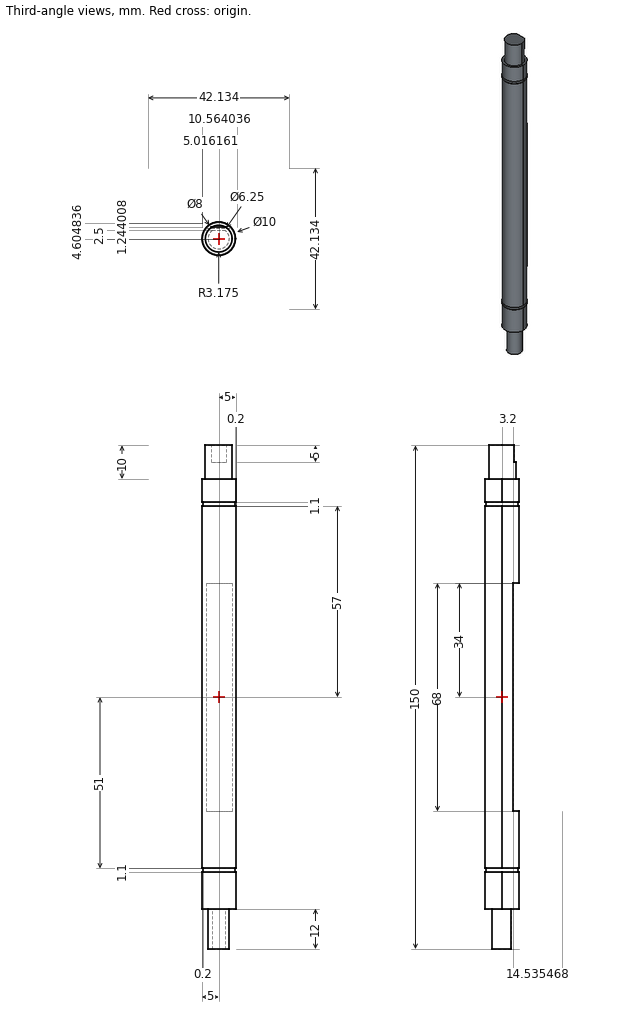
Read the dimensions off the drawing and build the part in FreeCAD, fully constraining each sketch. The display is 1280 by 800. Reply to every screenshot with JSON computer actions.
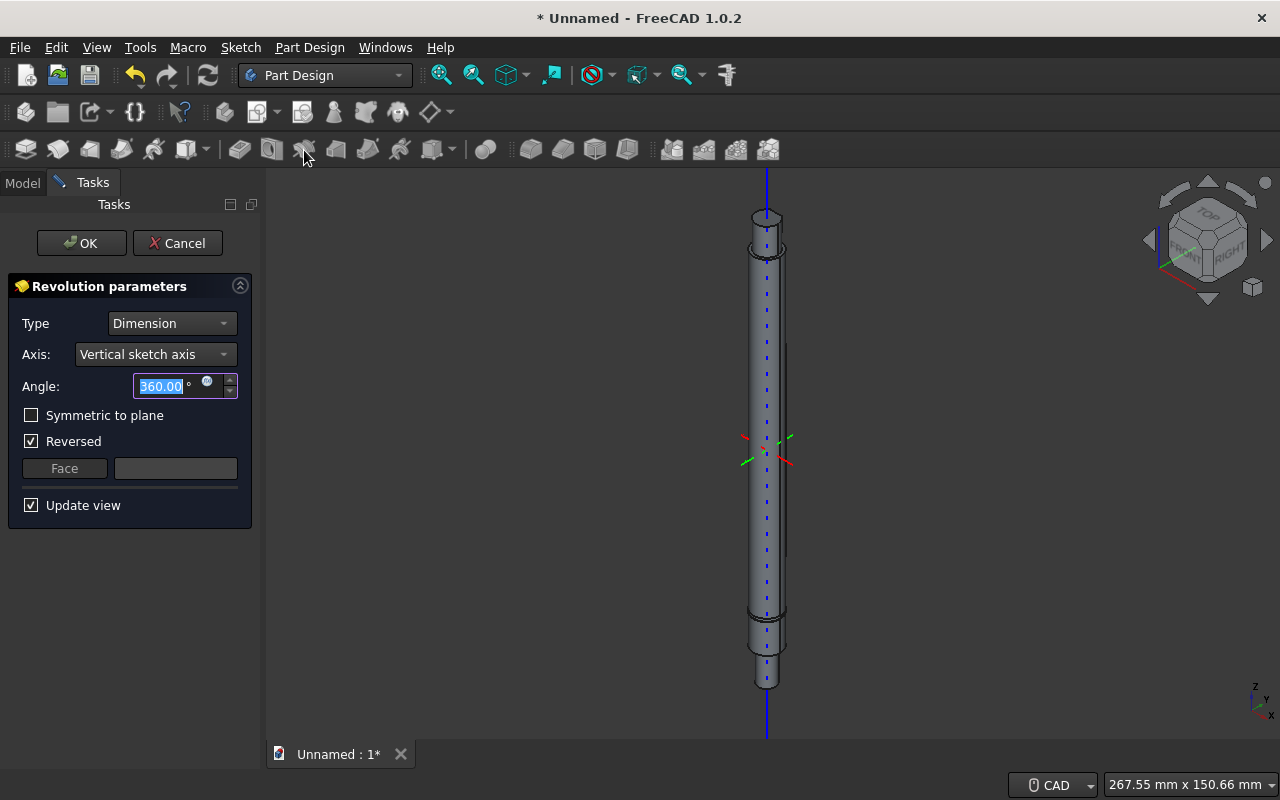
{"action": "left_click", "coordinate": [82, 243]}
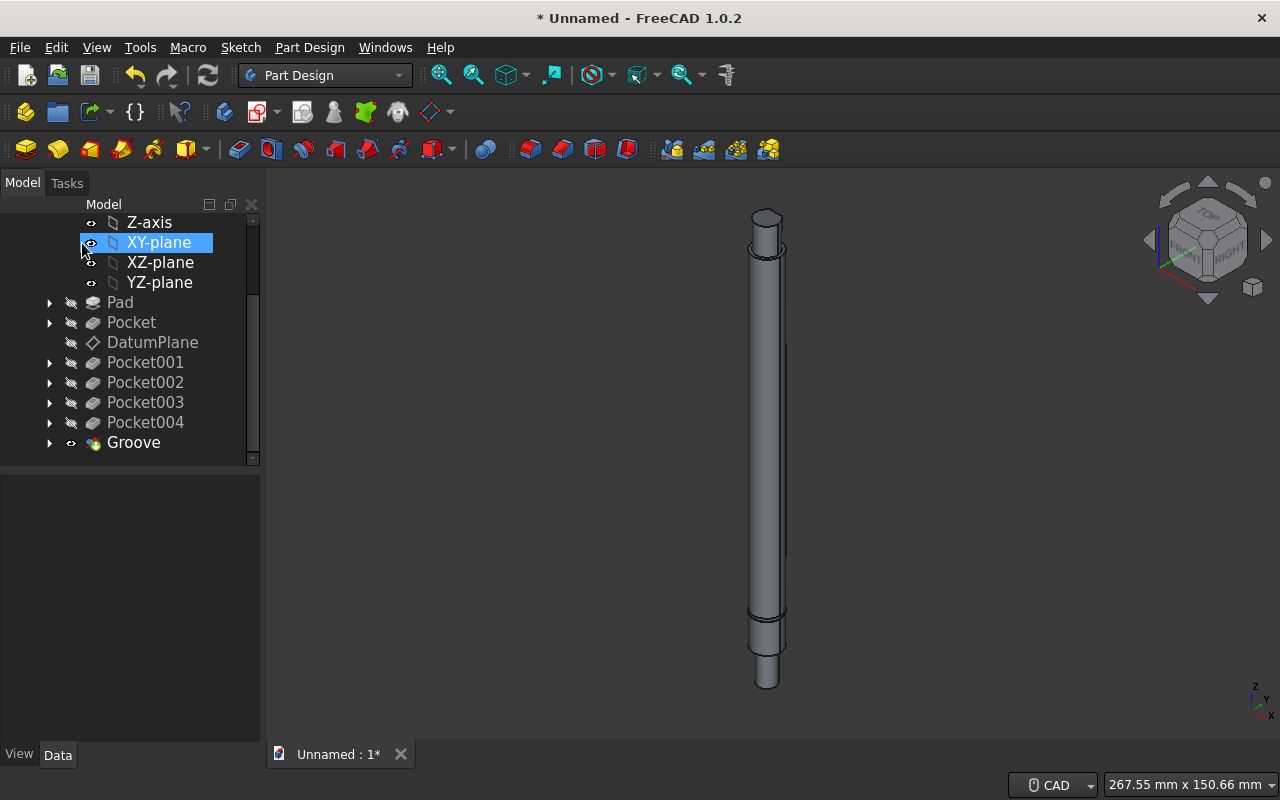
{"action": "left_click", "coordinate": [258, 112]}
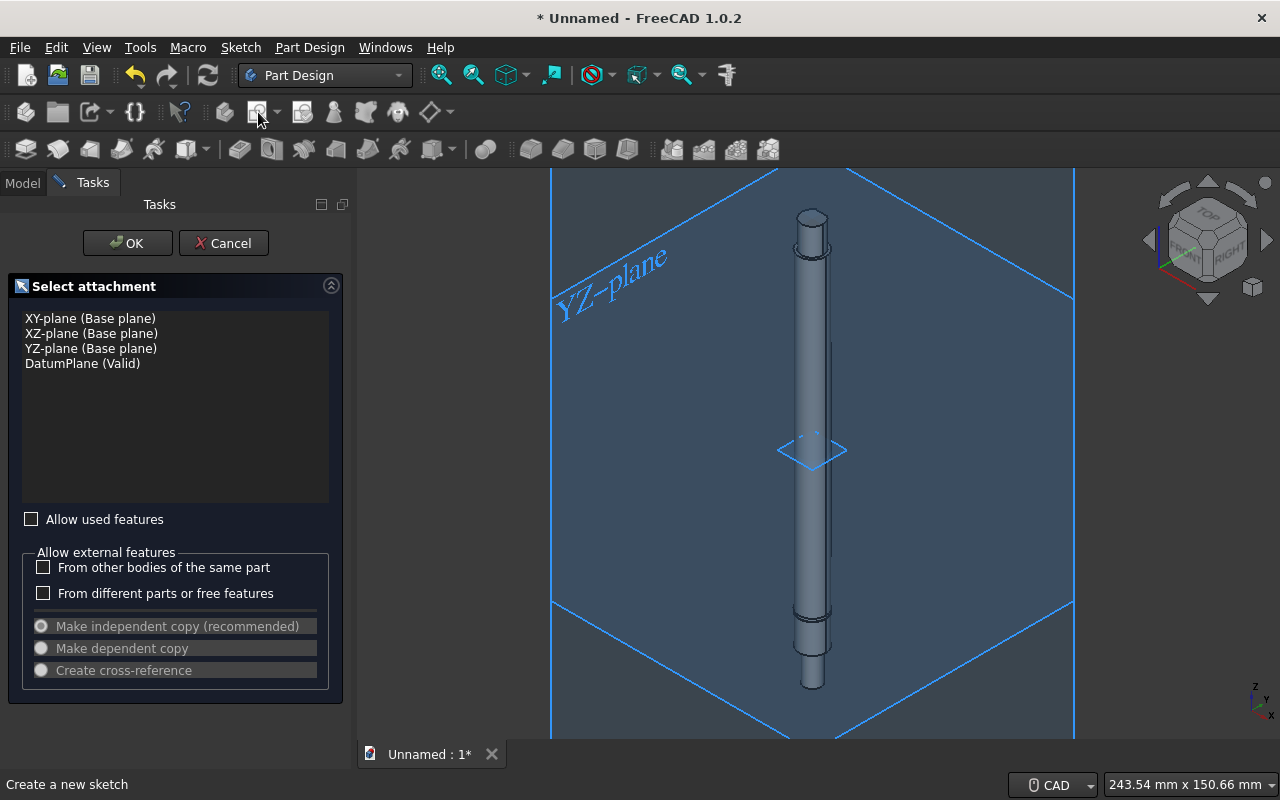
{"action": "left_click", "coordinate": [82, 334]}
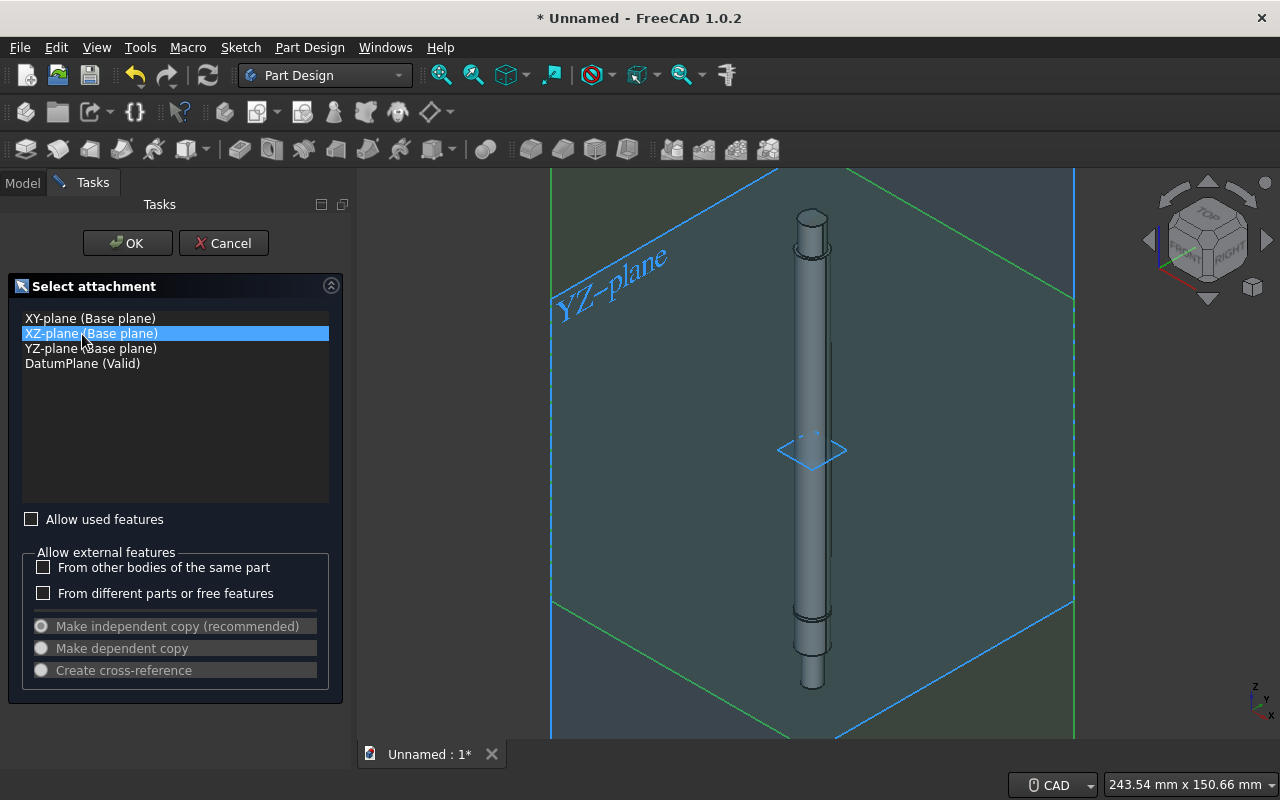
{"action": "left_click", "coordinate": [128, 243]}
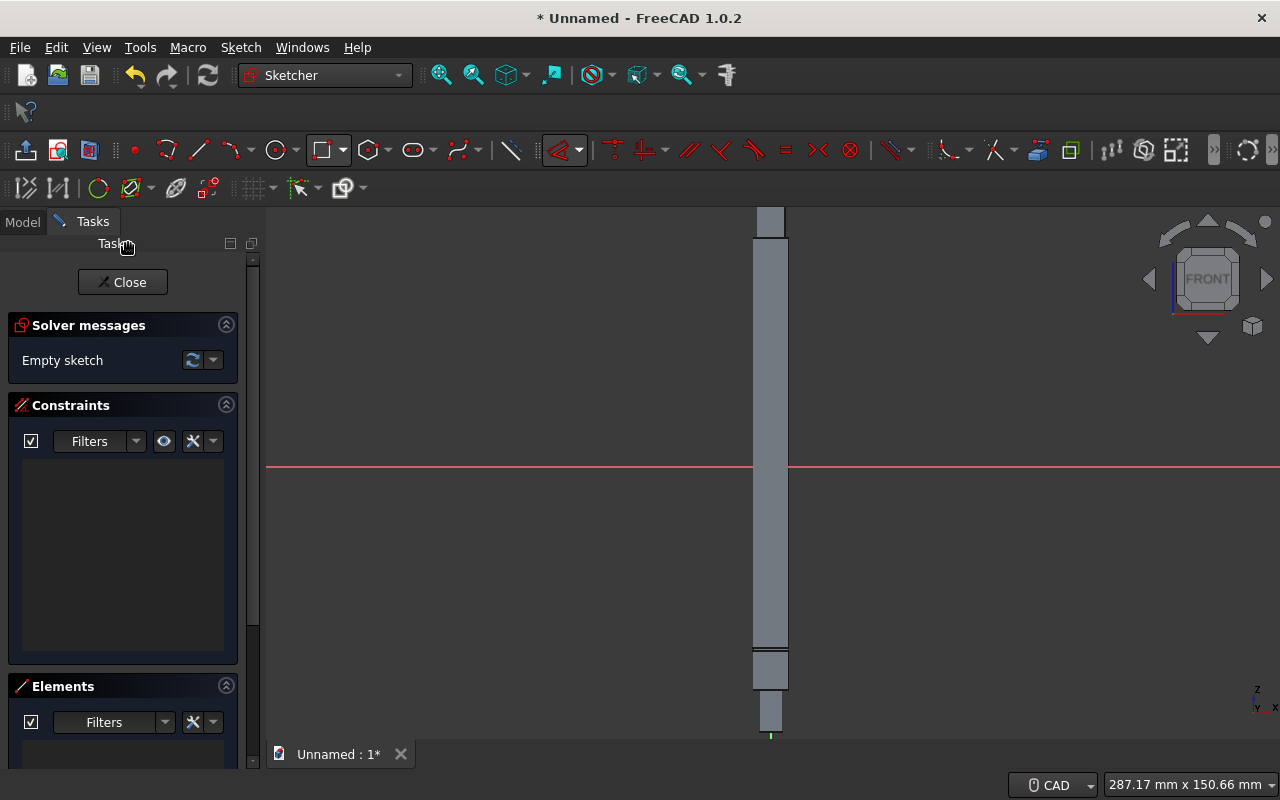
{"action": "left_click", "coordinate": [90, 150]}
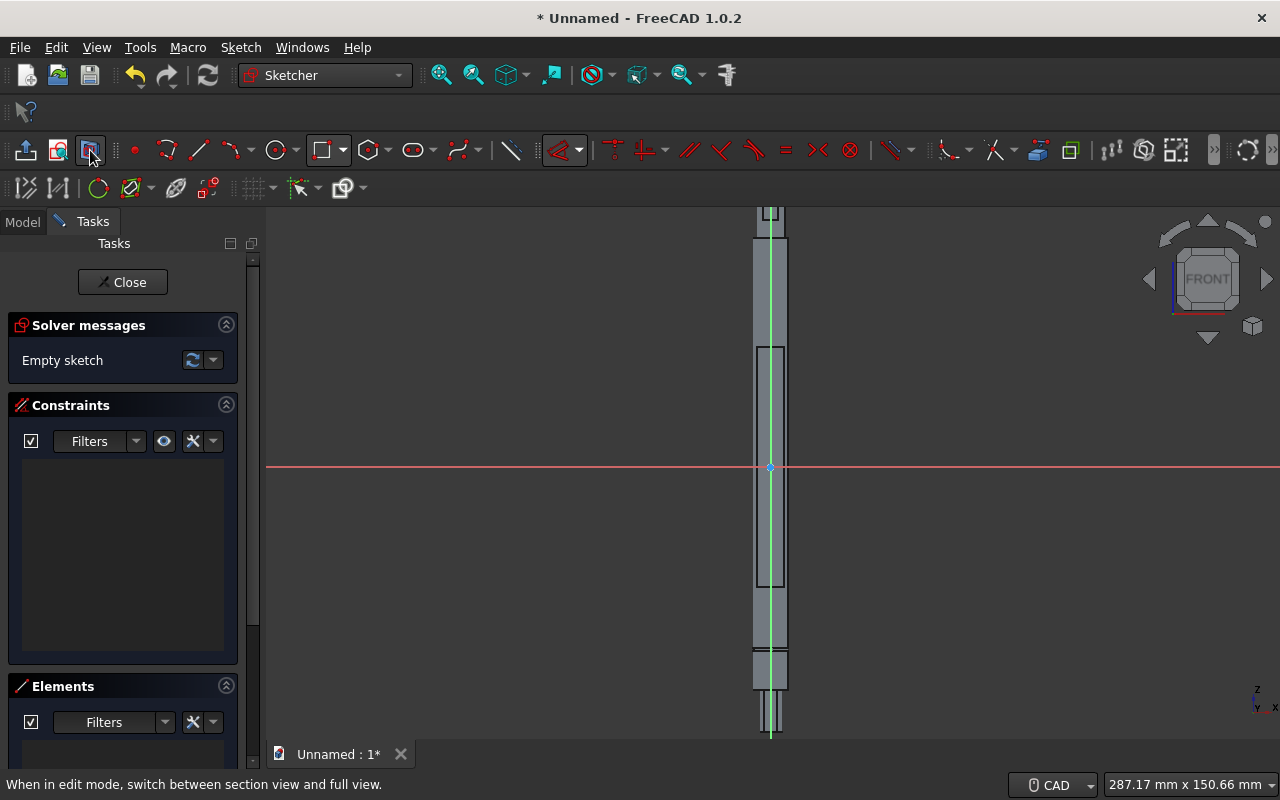
{"action": "scroll", "coordinate": [792, 253], "scroll_direction": "up", "scroll_amount": 15}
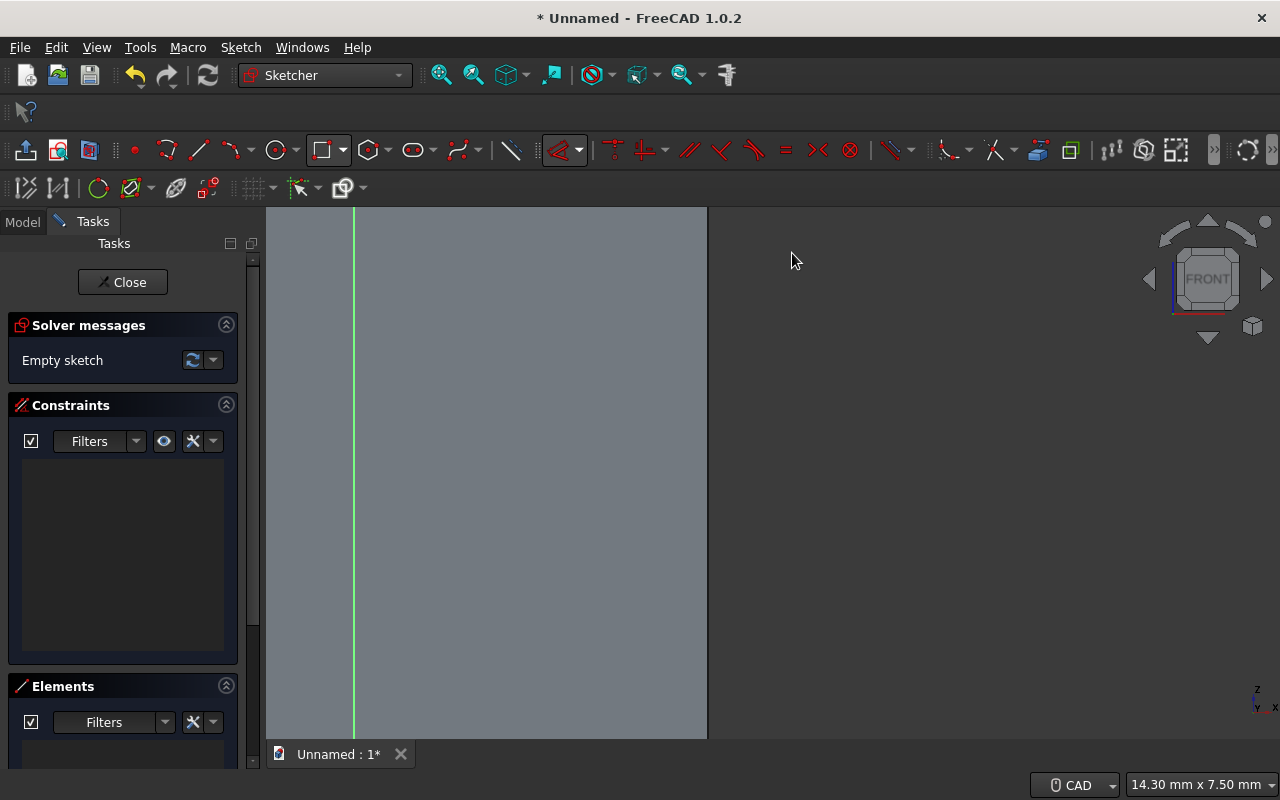
{"action": "scroll", "coordinate": [700, 478], "scroll_direction": "up", "scroll_amount": 7}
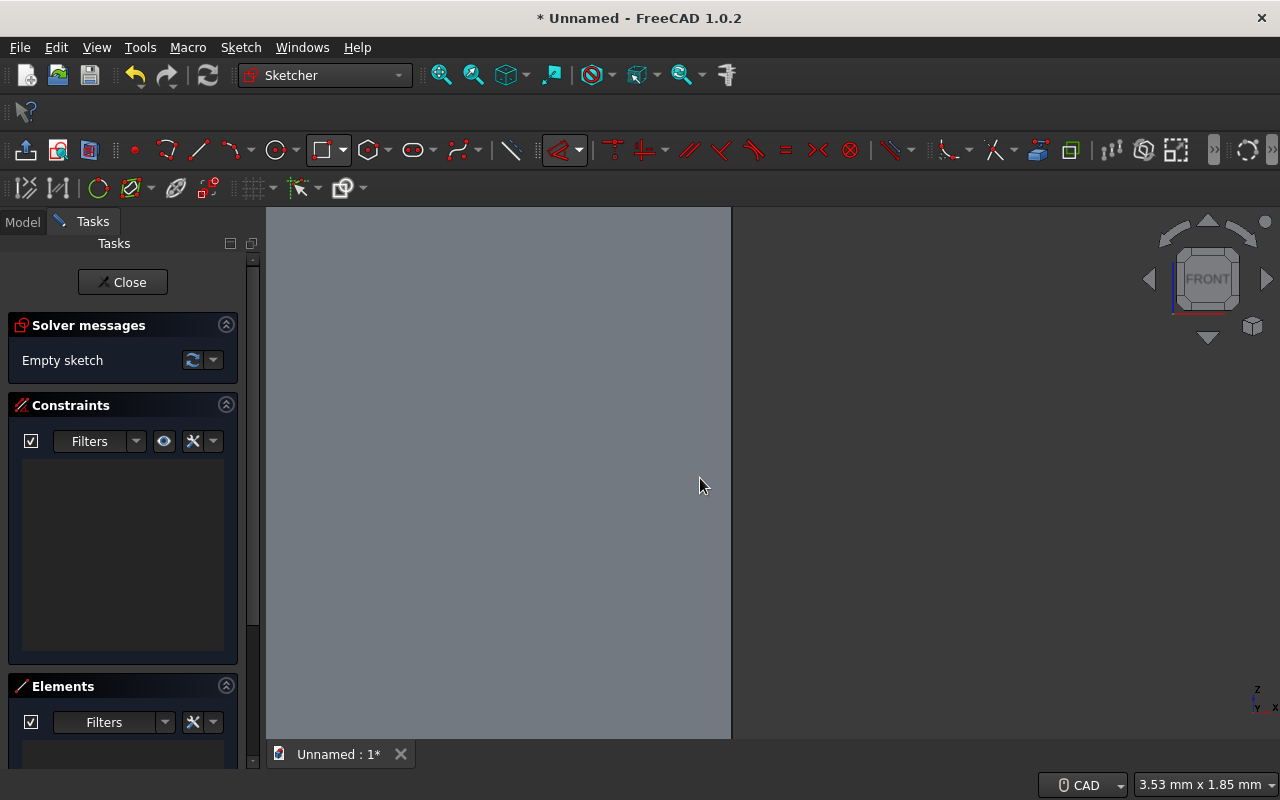
{"action": "left_click", "coordinate": [322, 150]}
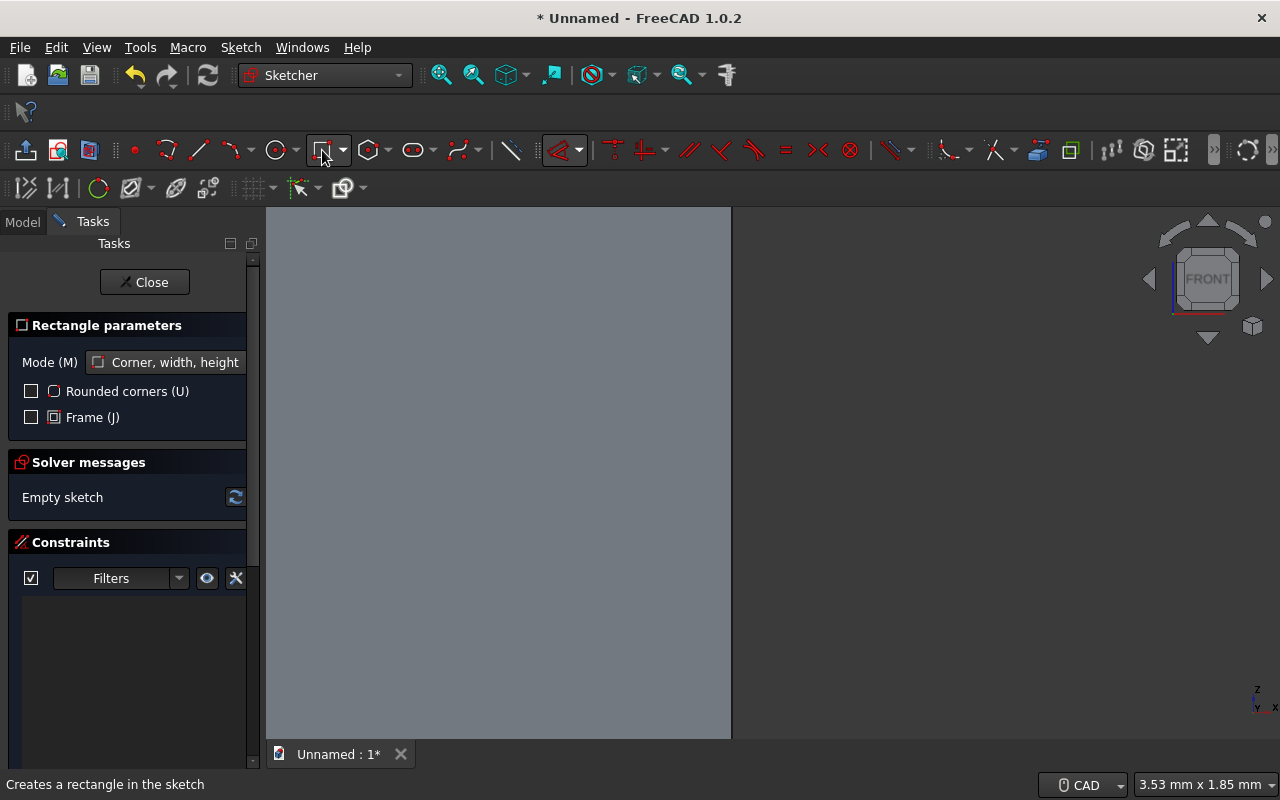
{"action": "left_click", "coordinate": [675, 314]}
{"action": "left_click", "coordinate": [732, 630]}
{"action": "key", "text": "Escape"}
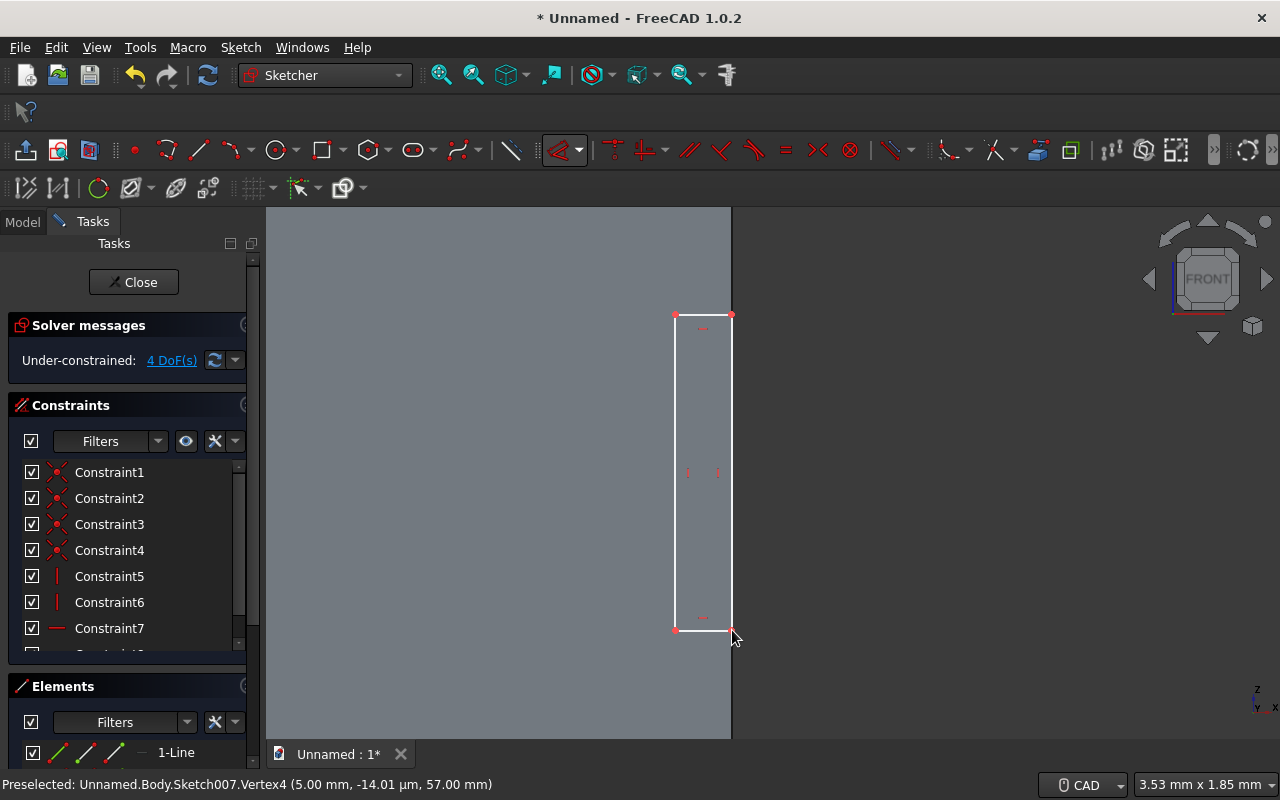
{"action": "left_click", "coordinate": [732, 631]}